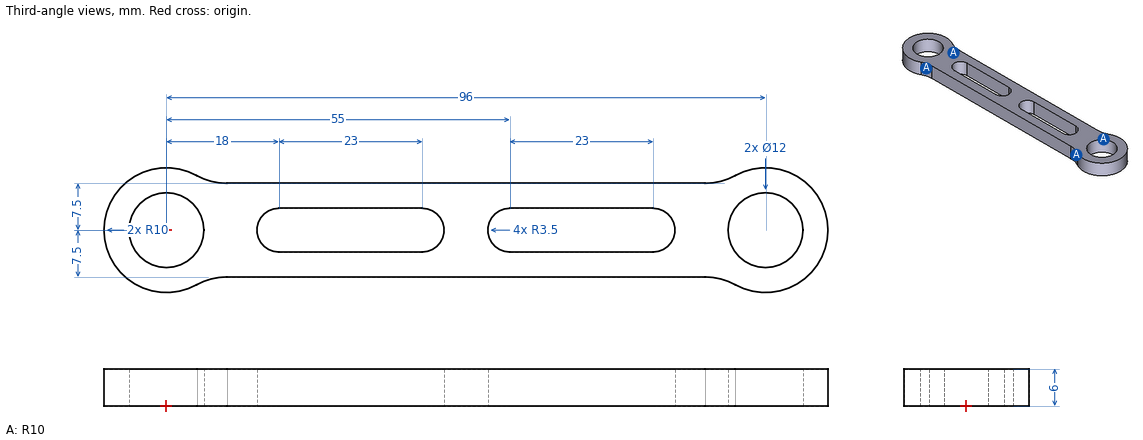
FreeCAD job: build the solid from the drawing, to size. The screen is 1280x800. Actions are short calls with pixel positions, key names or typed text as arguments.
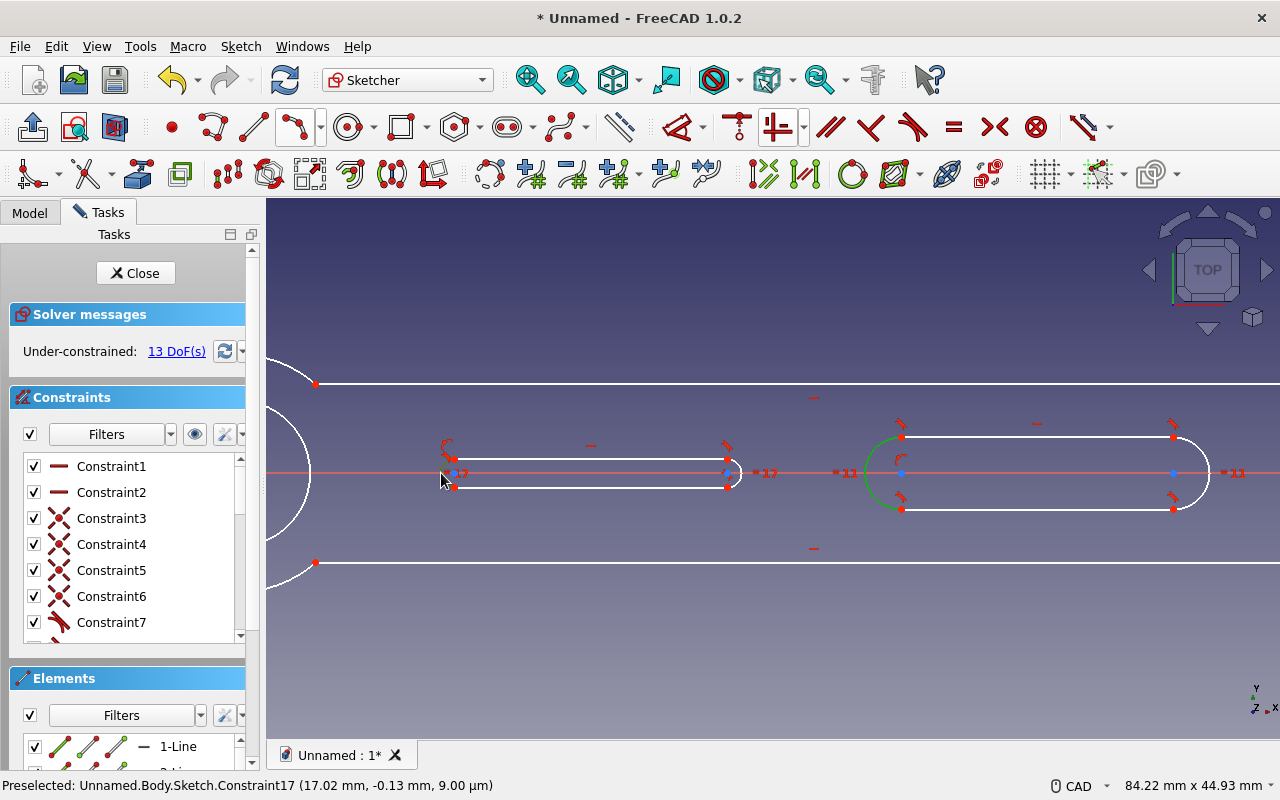
click(954, 128)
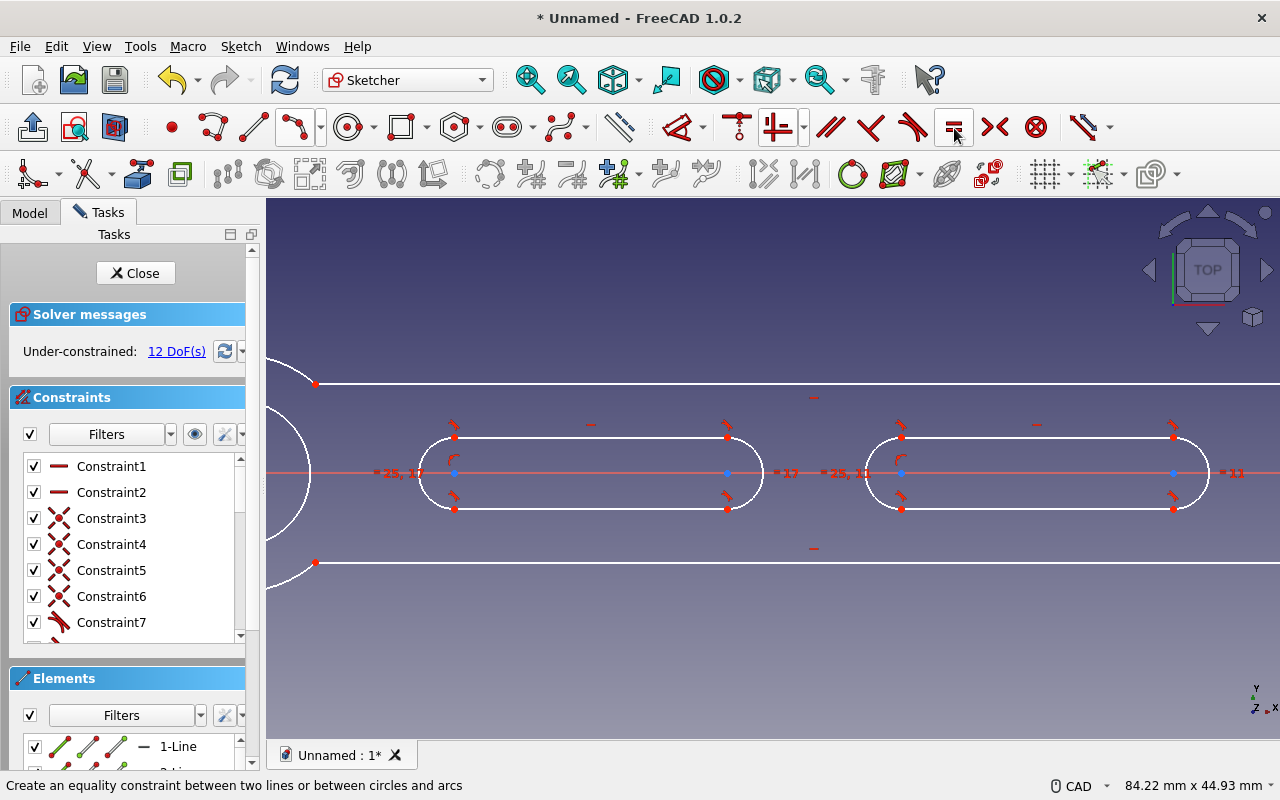
scroll(614, 464, down, 4)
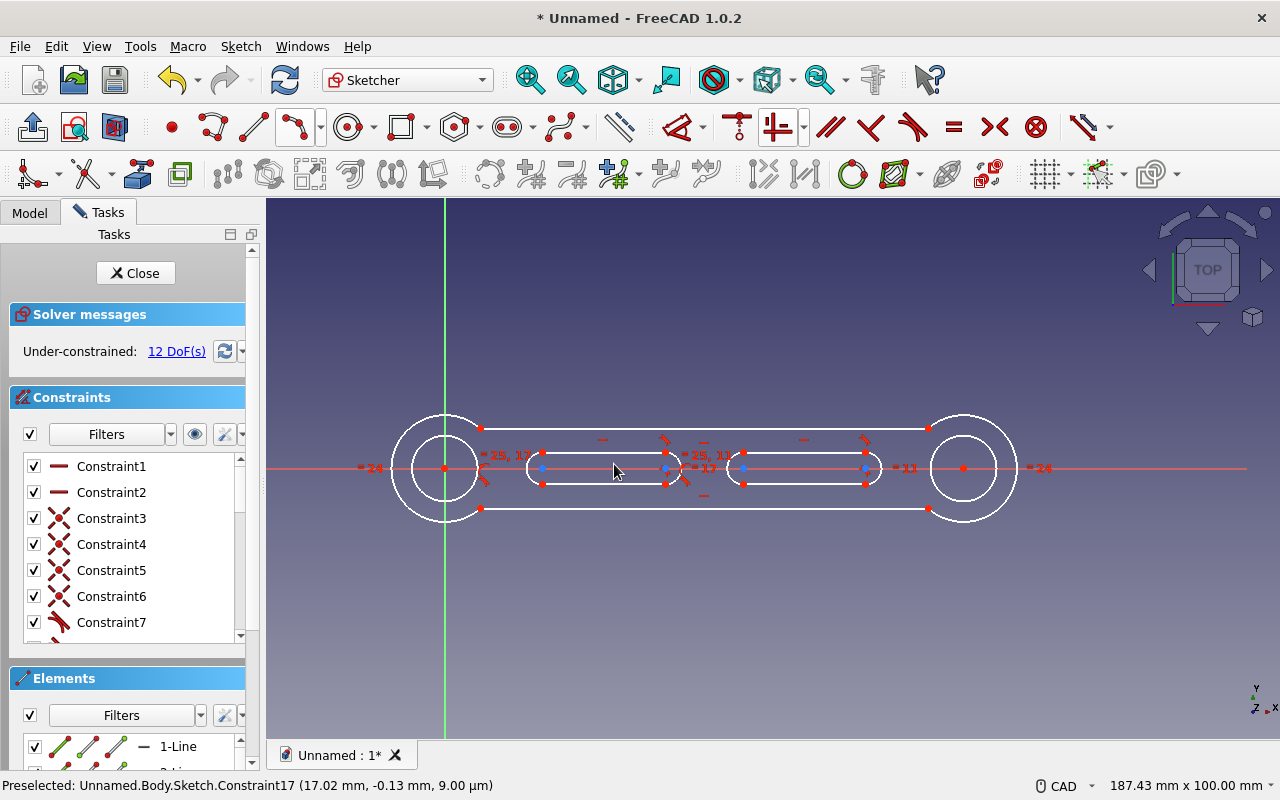
click(987, 445)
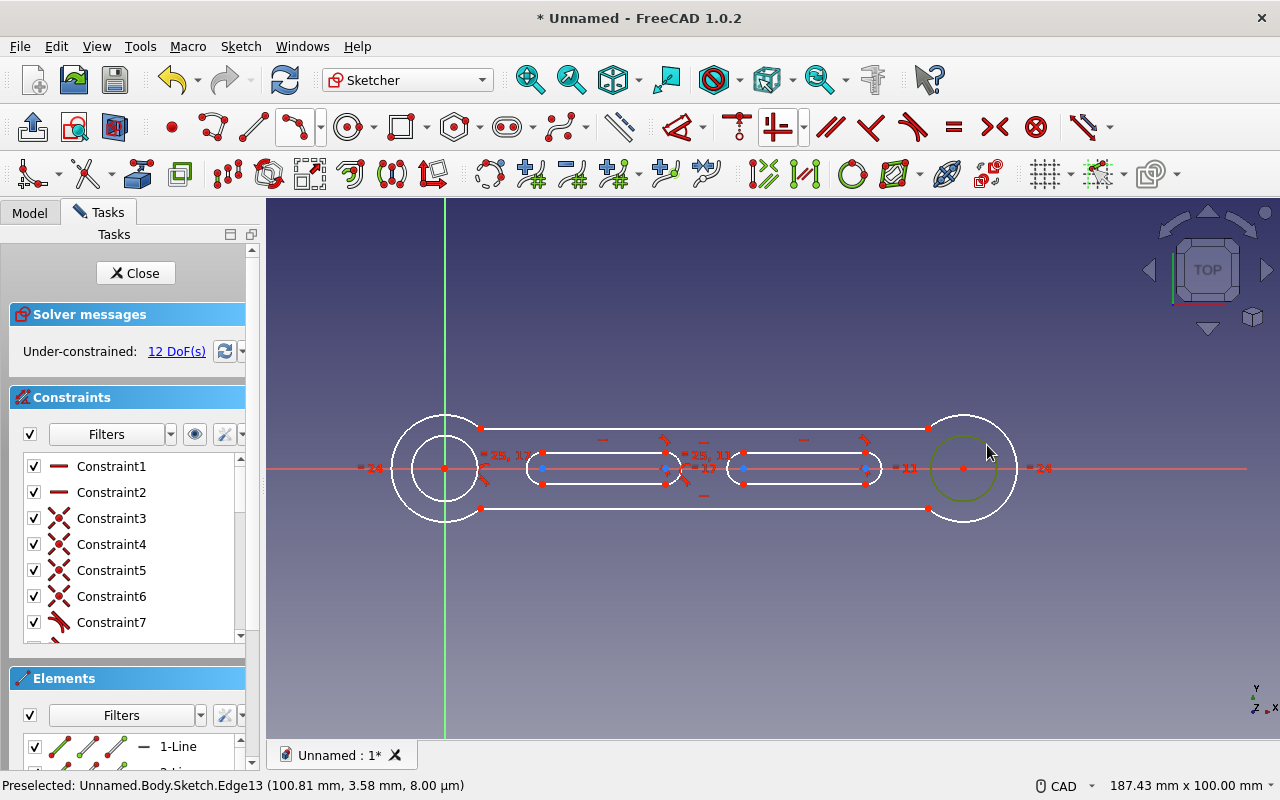
click(468, 445)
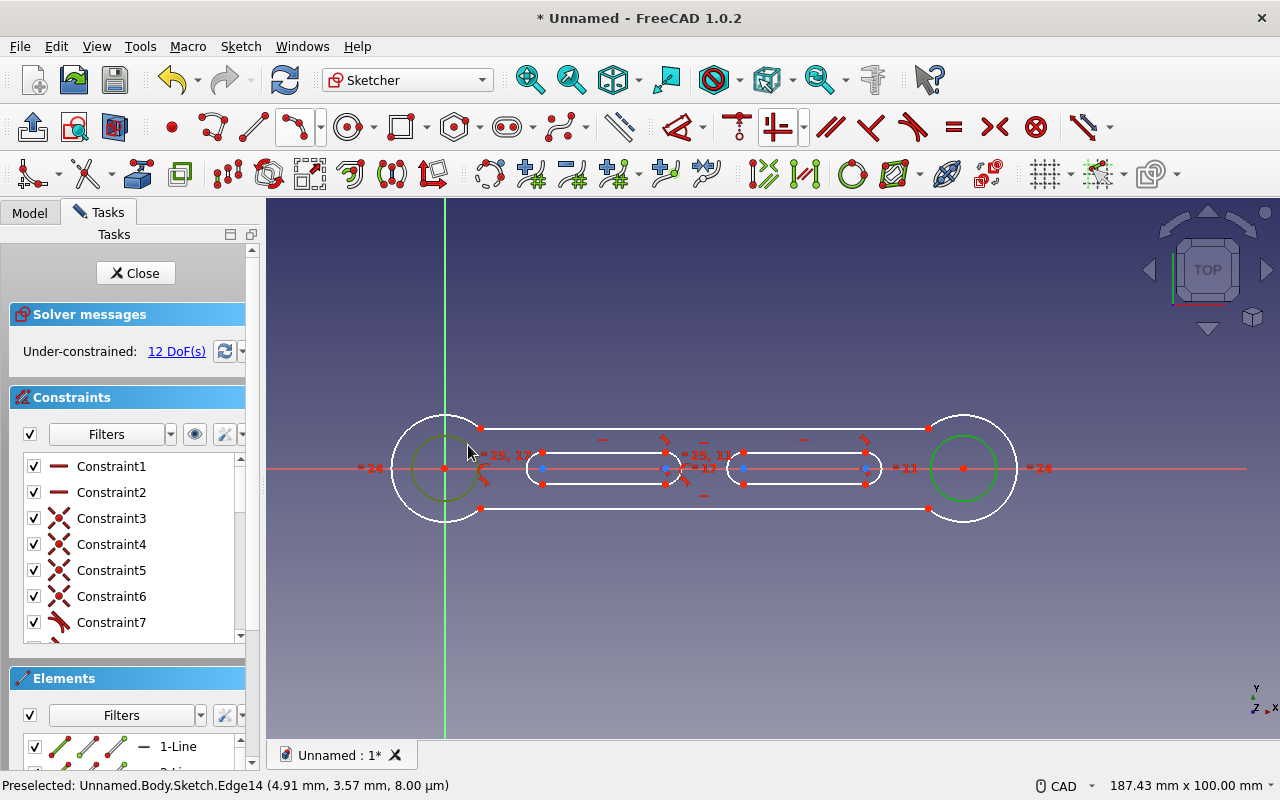
click(954, 128)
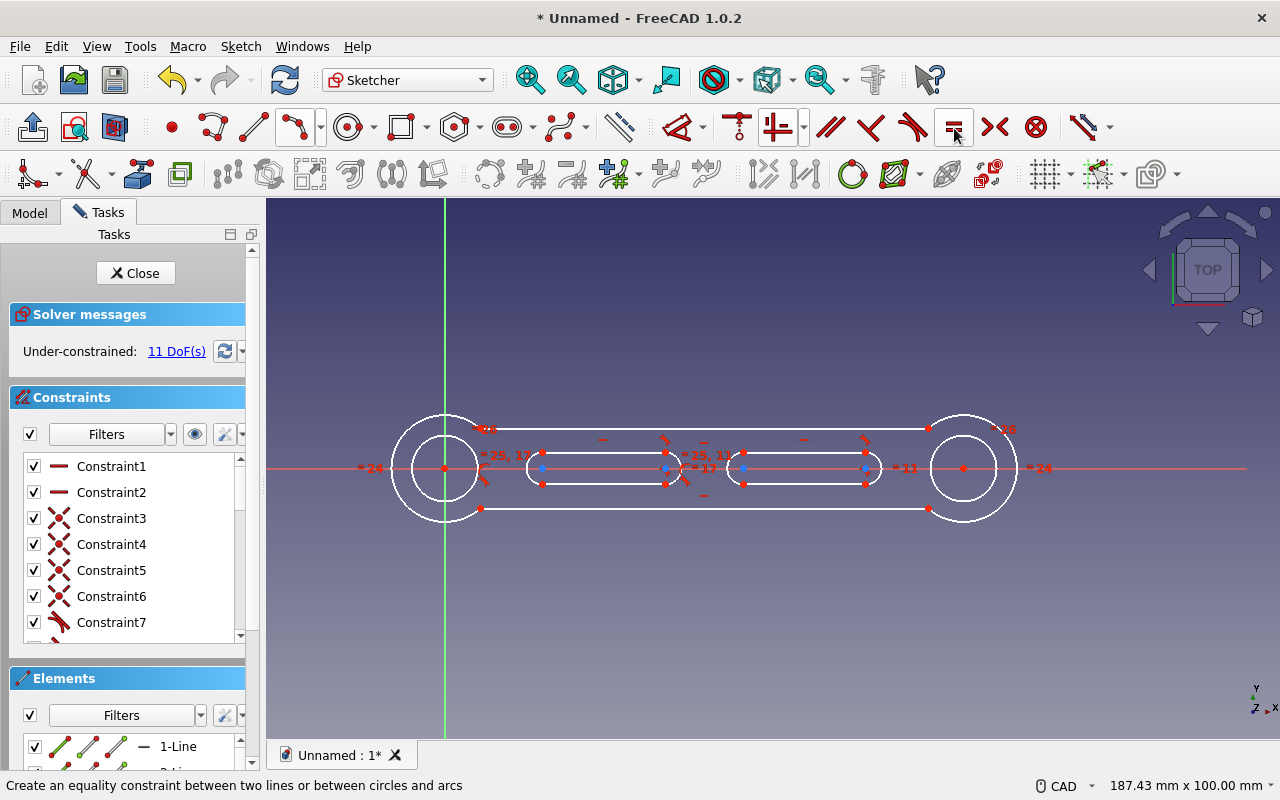
click(964, 469)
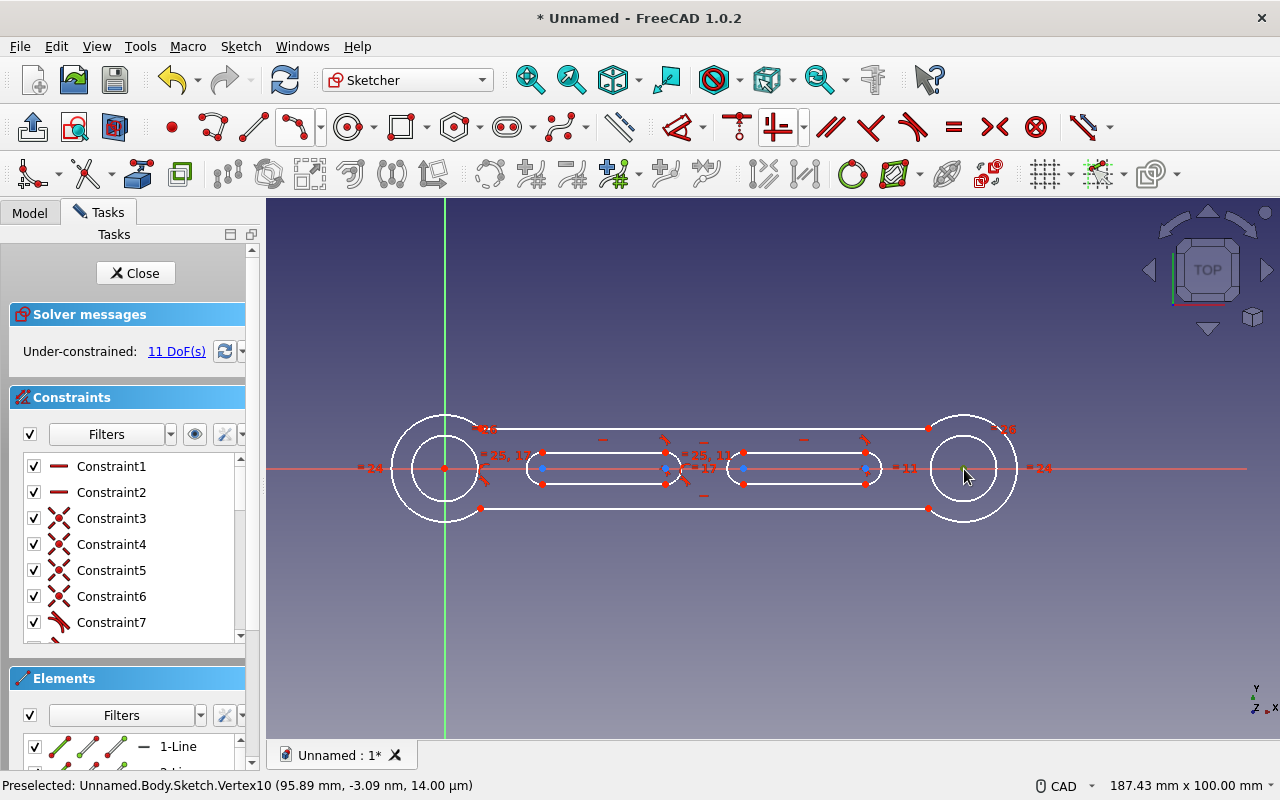
click(353, 469)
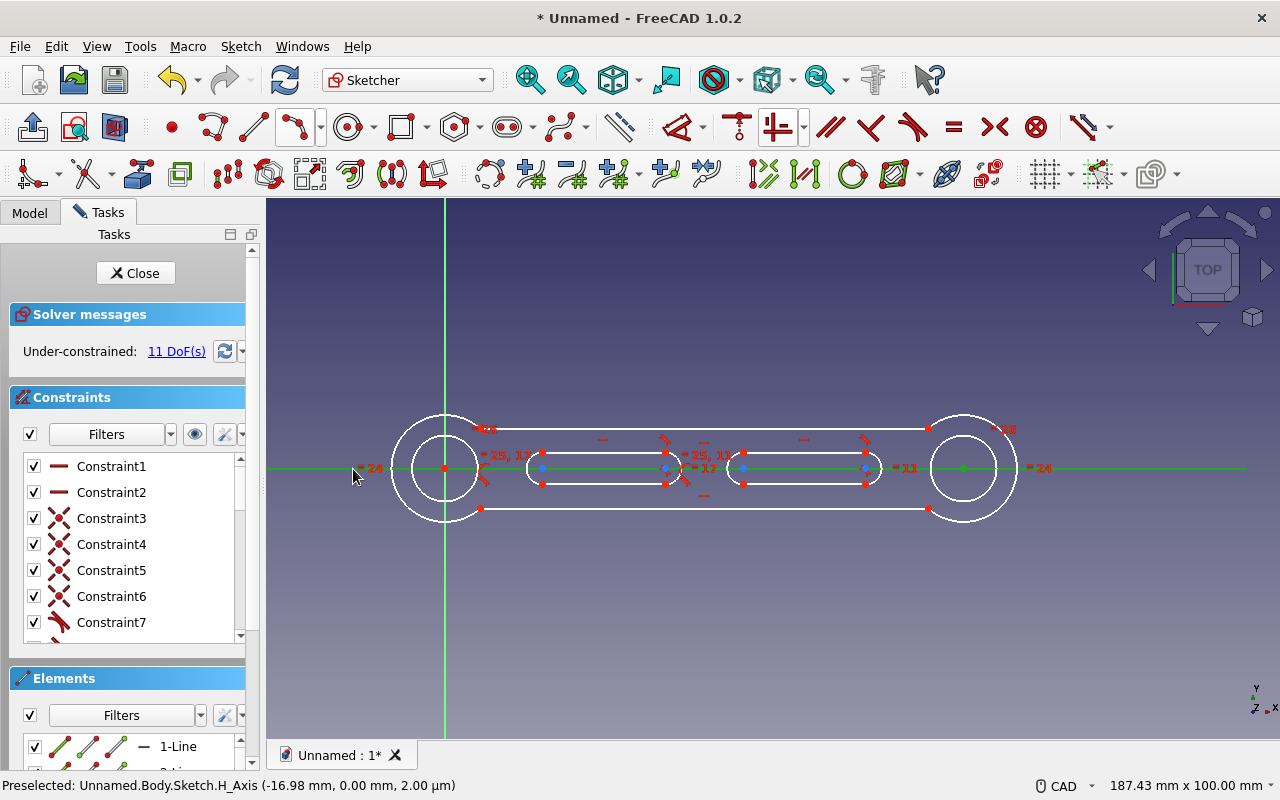
click(737, 128)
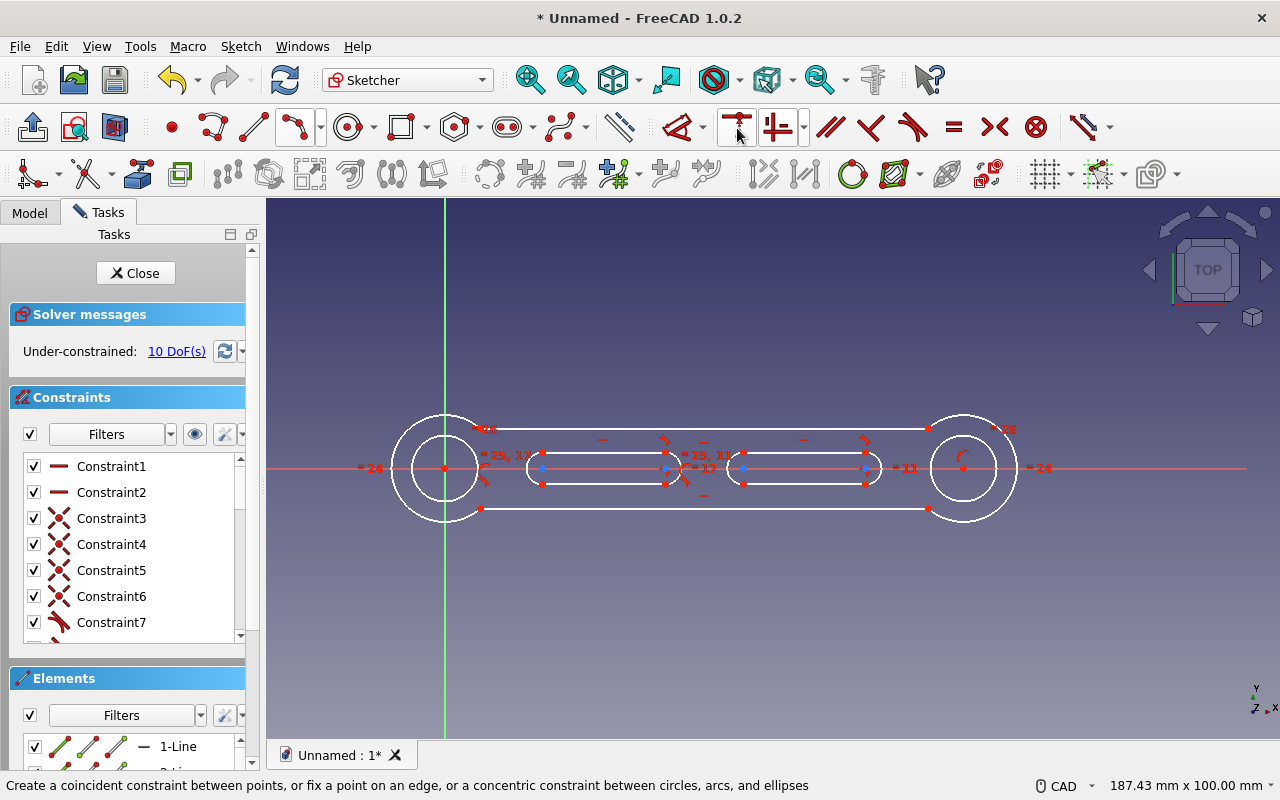
click(676, 128)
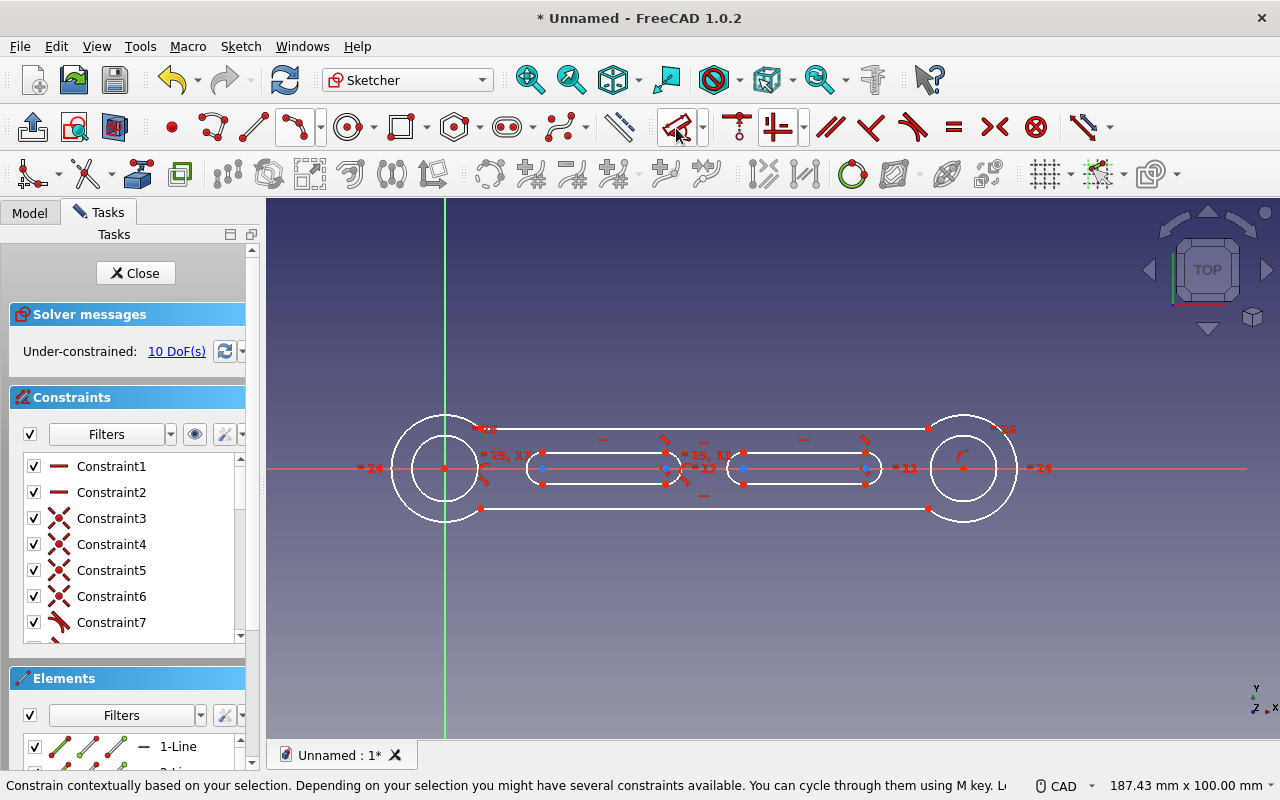
click(412, 426)
click(392, 401)